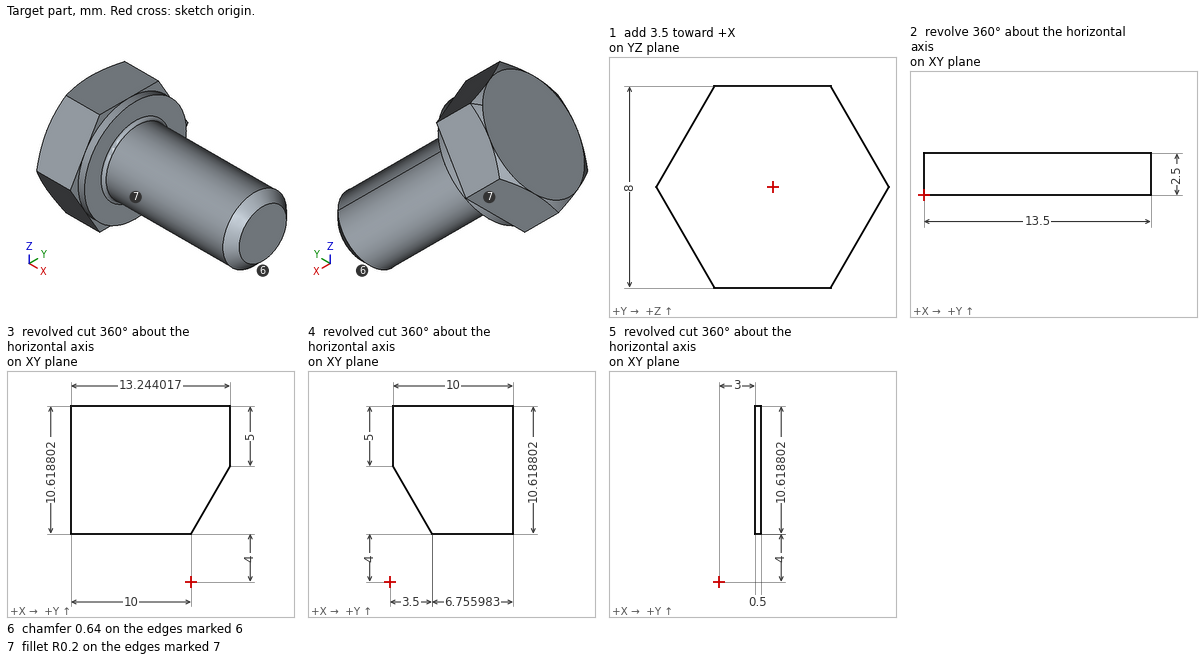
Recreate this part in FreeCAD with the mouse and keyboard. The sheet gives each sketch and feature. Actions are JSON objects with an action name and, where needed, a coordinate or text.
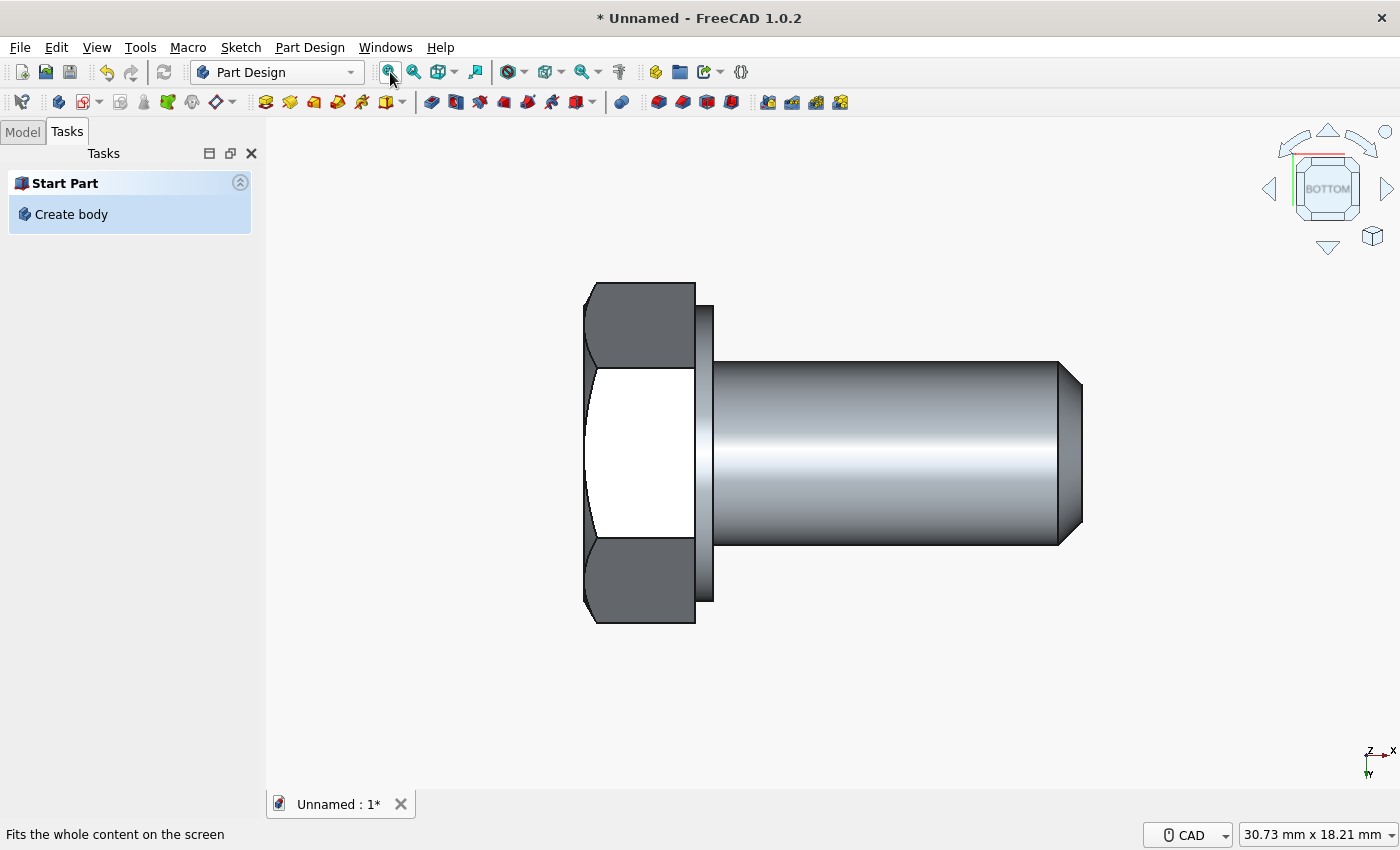
{"action": "key", "text": "4"}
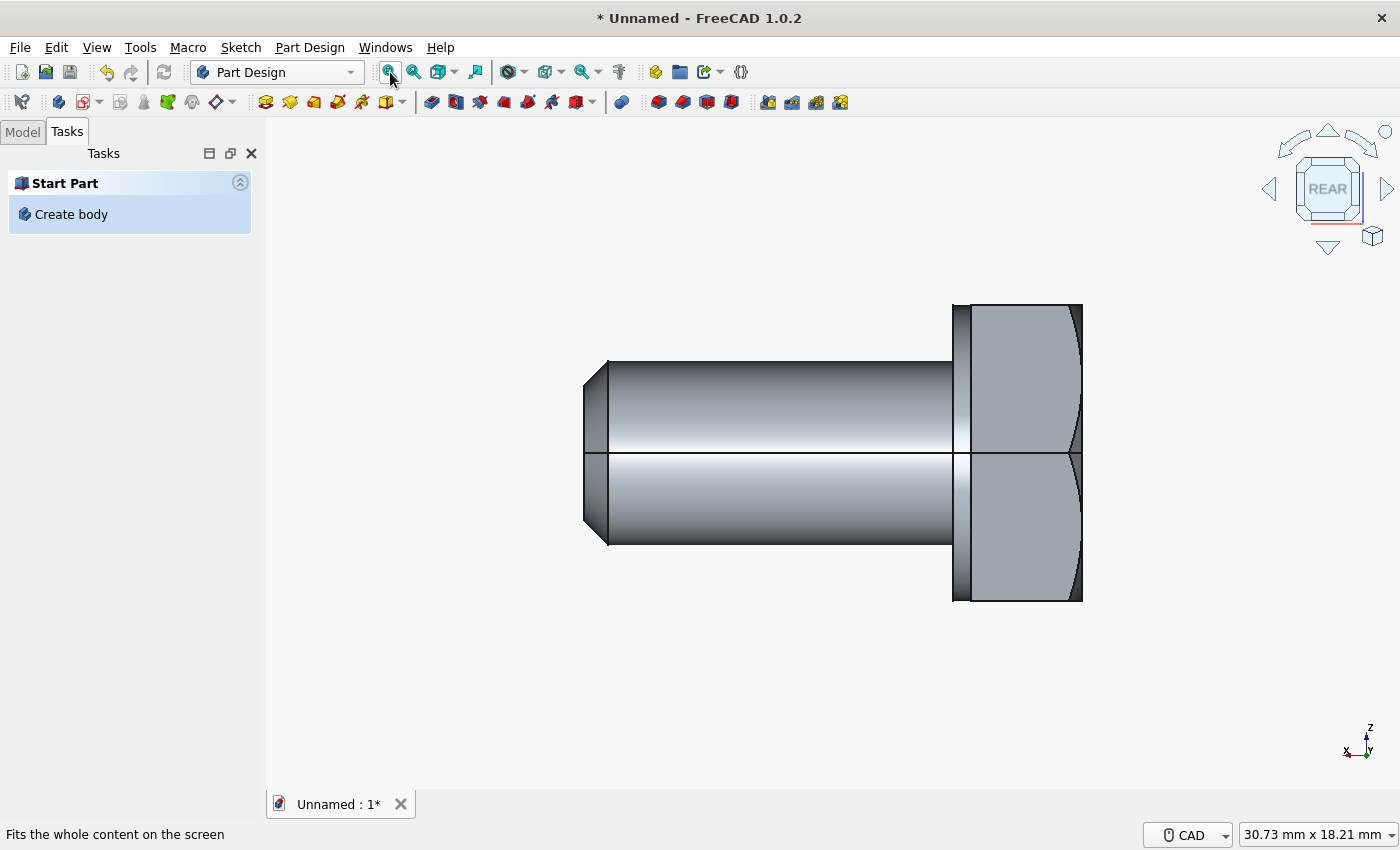
{"action": "left_click", "coordinate": [390, 72]}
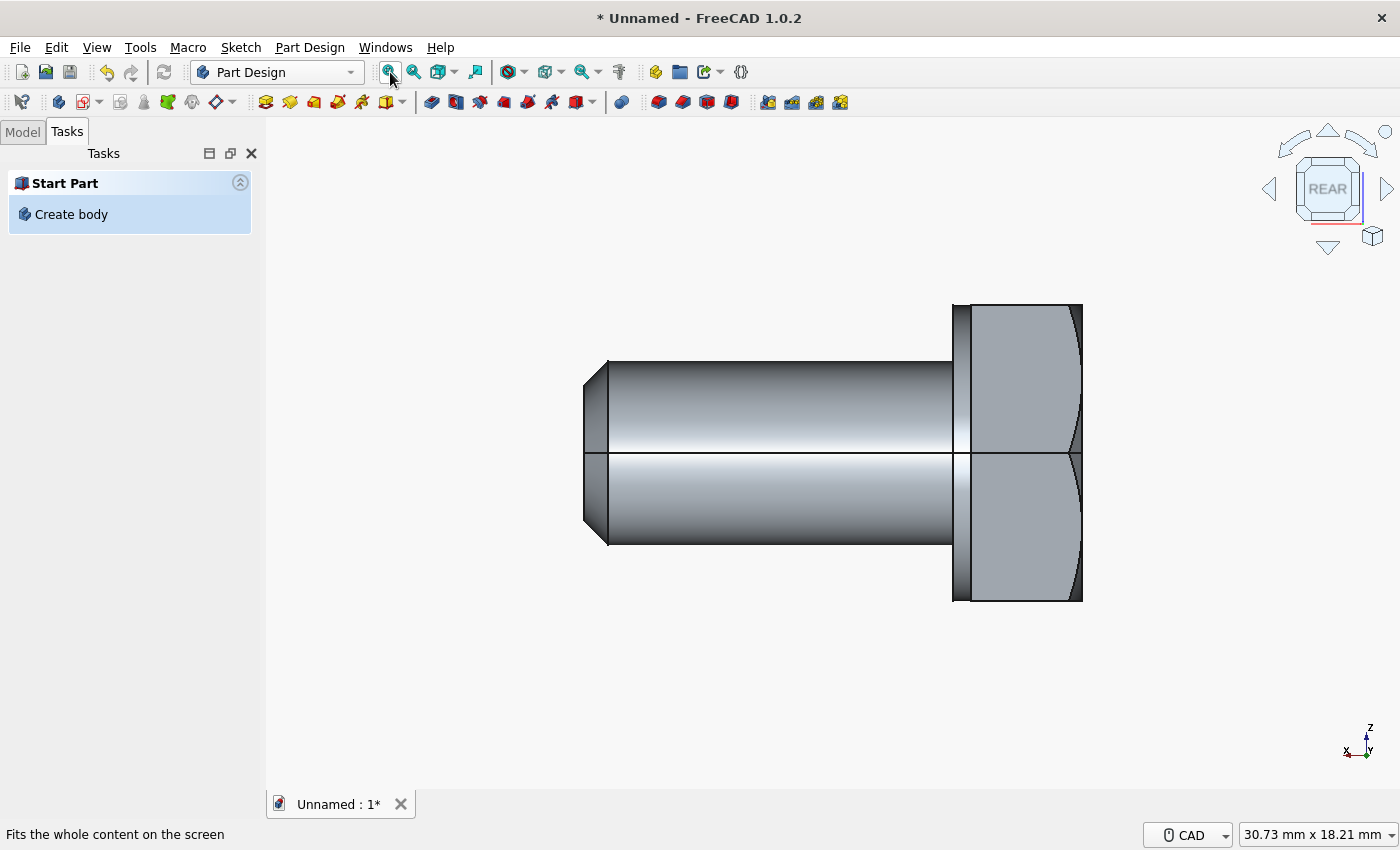
{"action": "key", "text": "6"}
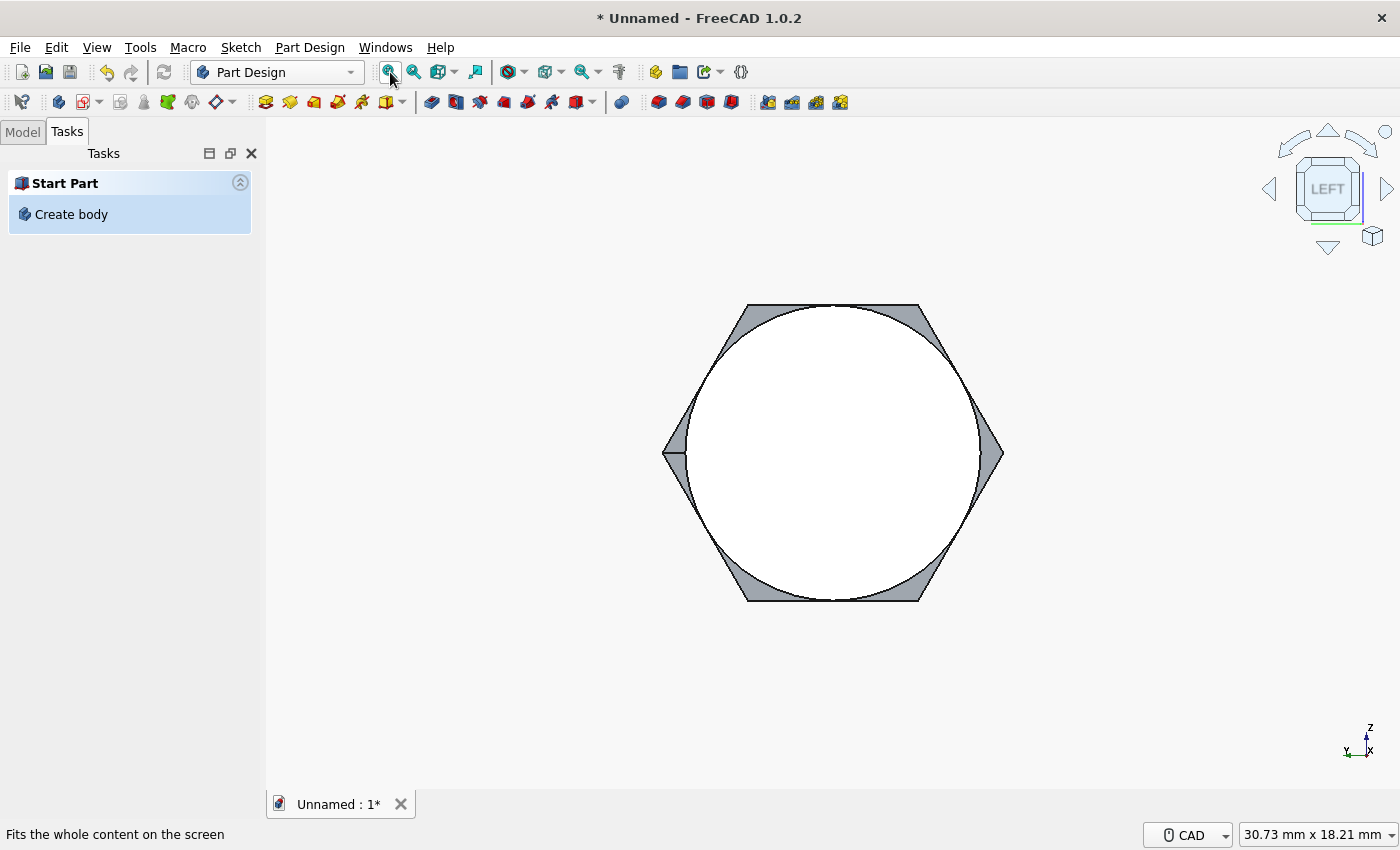
{"action": "left_click", "coordinate": [390, 72]}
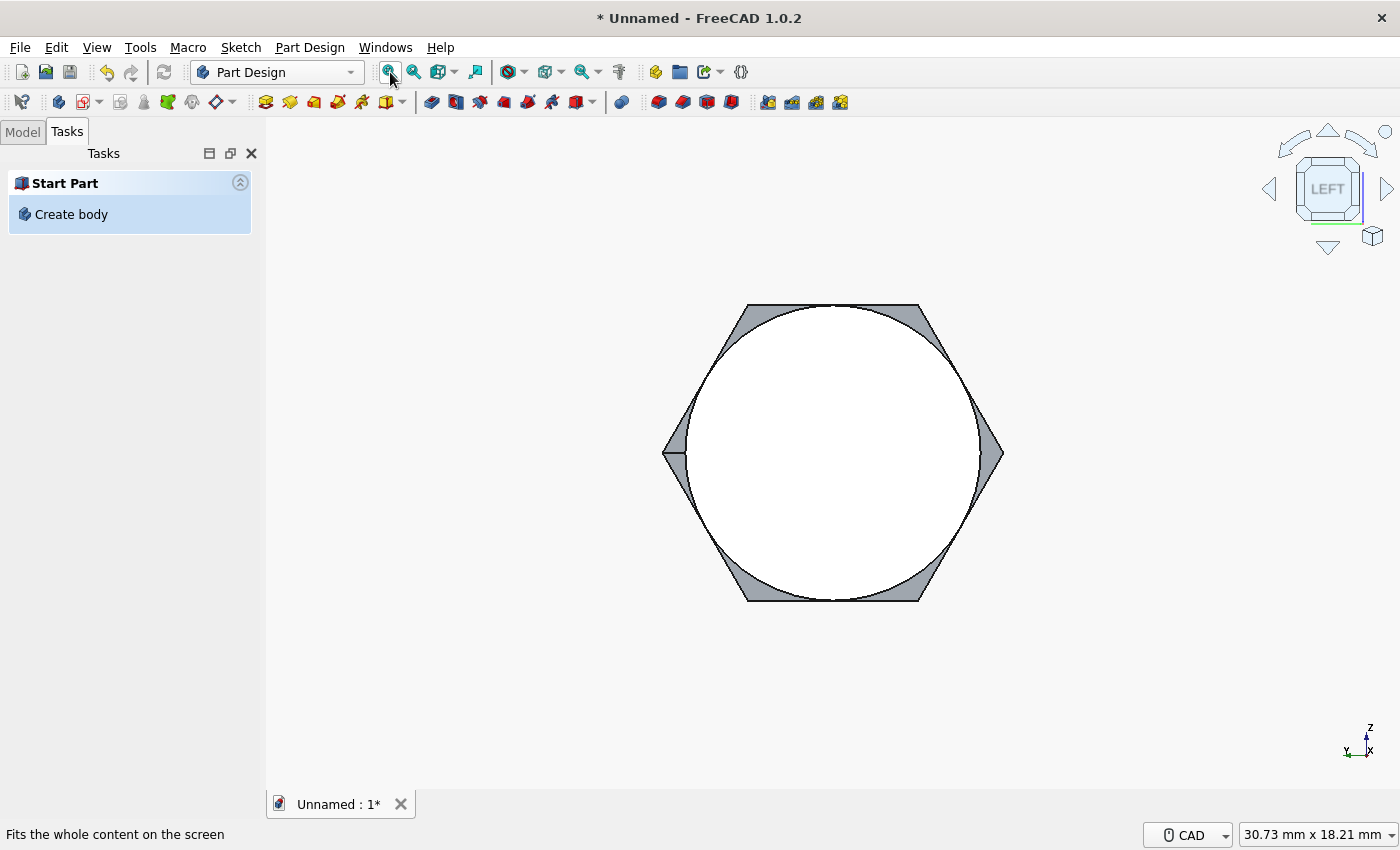
{"action": "key", "text": "v 3"}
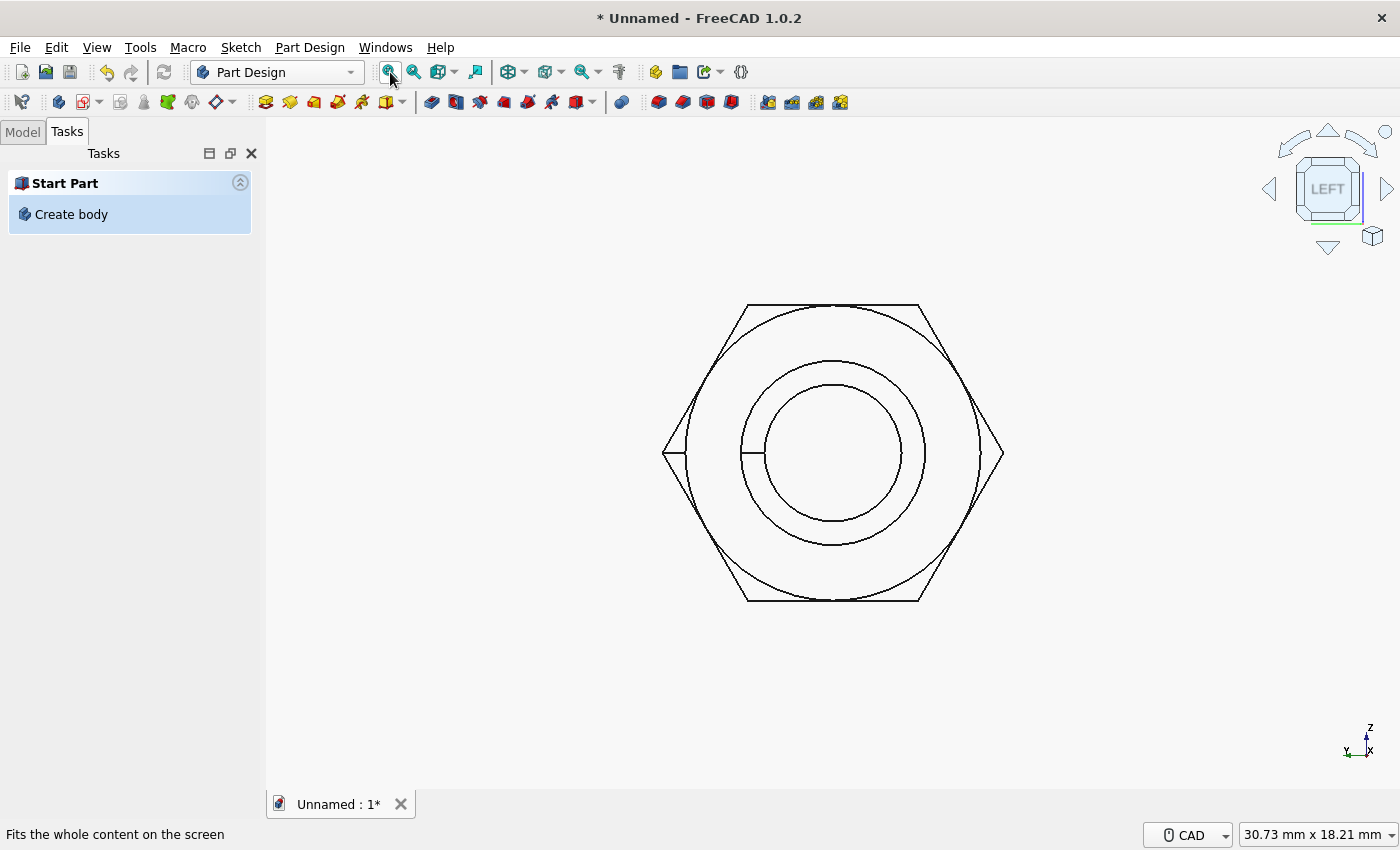
{"action": "key", "text": "0"}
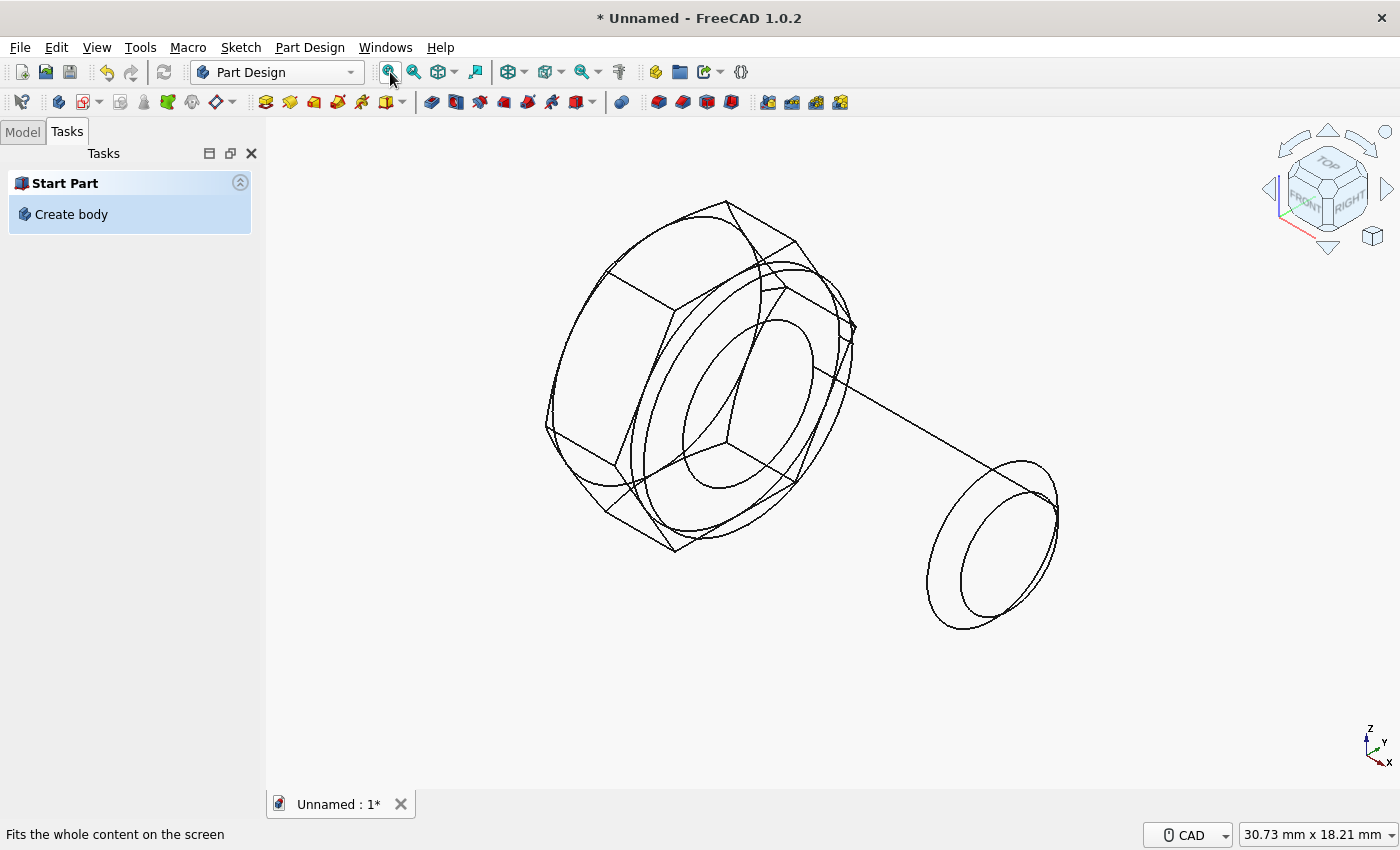
{"action": "left_click", "coordinate": [683, 441]}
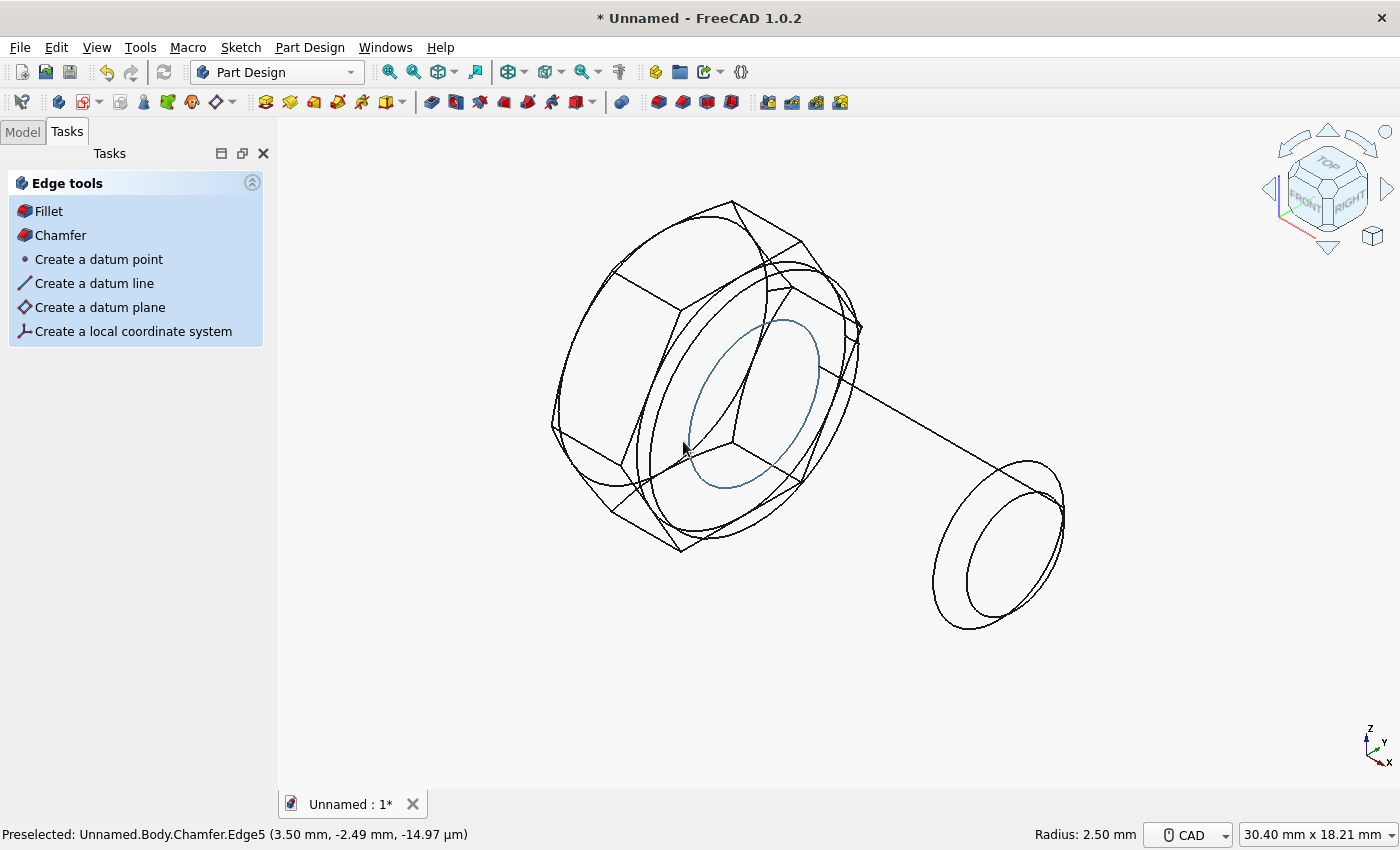
{"action": "key", "text": "v 1"}